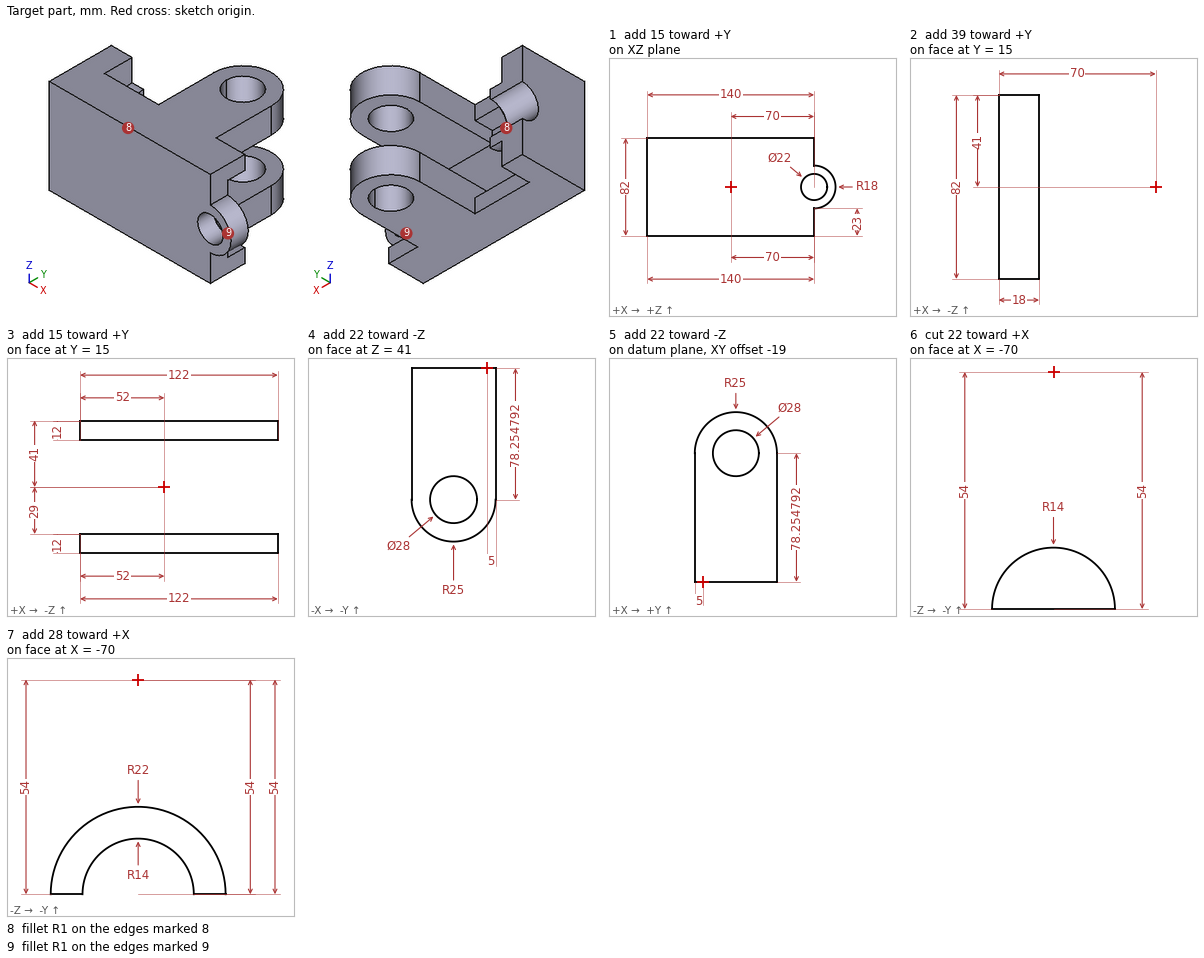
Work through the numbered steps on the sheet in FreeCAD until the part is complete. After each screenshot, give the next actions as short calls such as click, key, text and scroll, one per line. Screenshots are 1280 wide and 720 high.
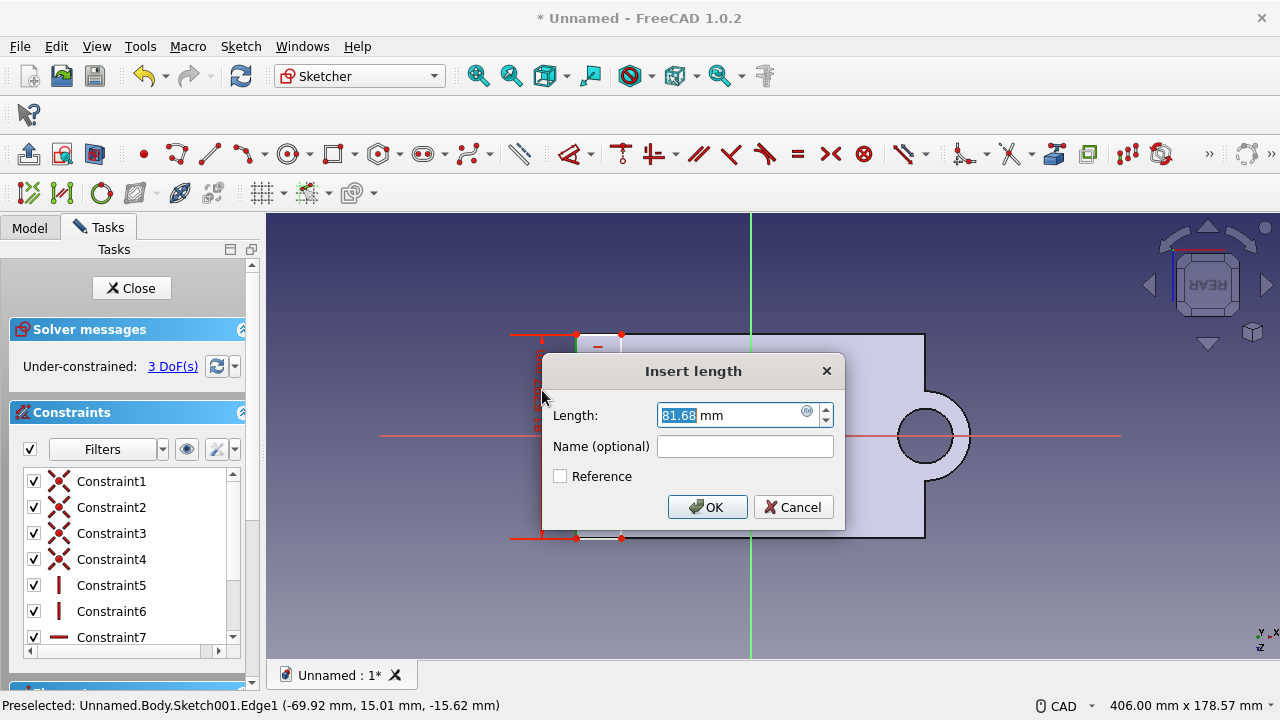
text(82)
key(Return)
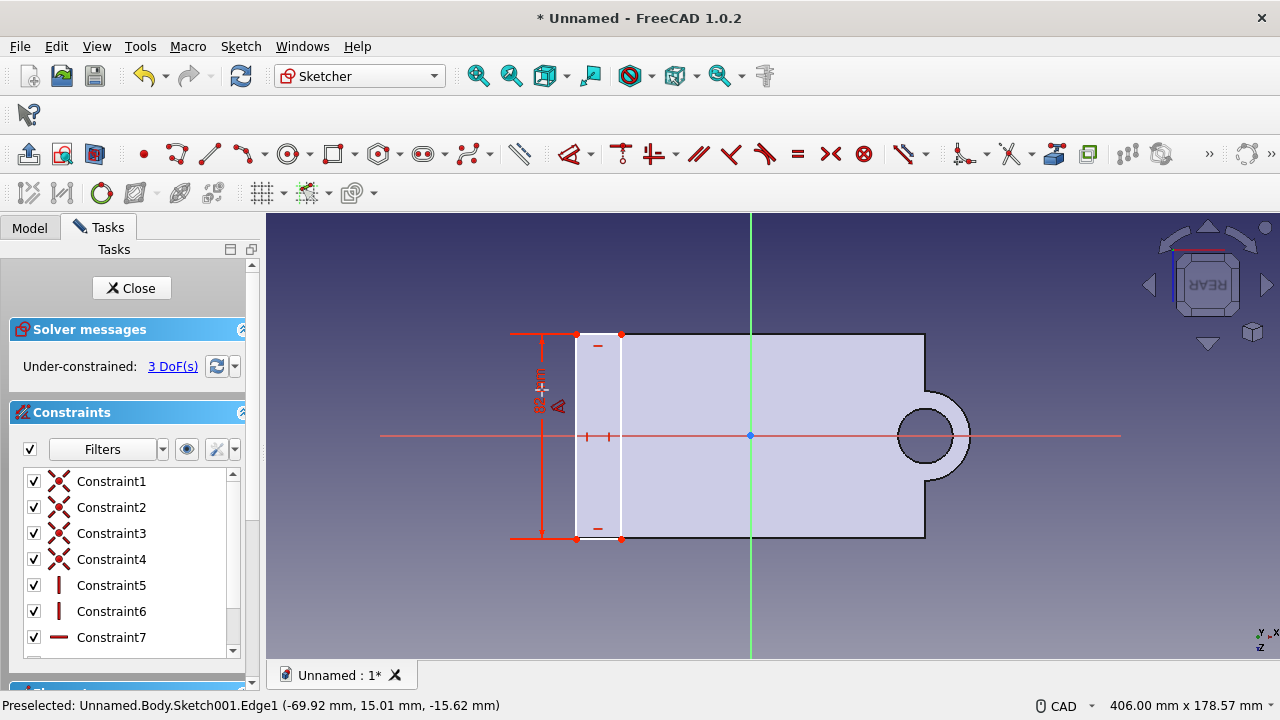
click(589, 539)
click(598, 573)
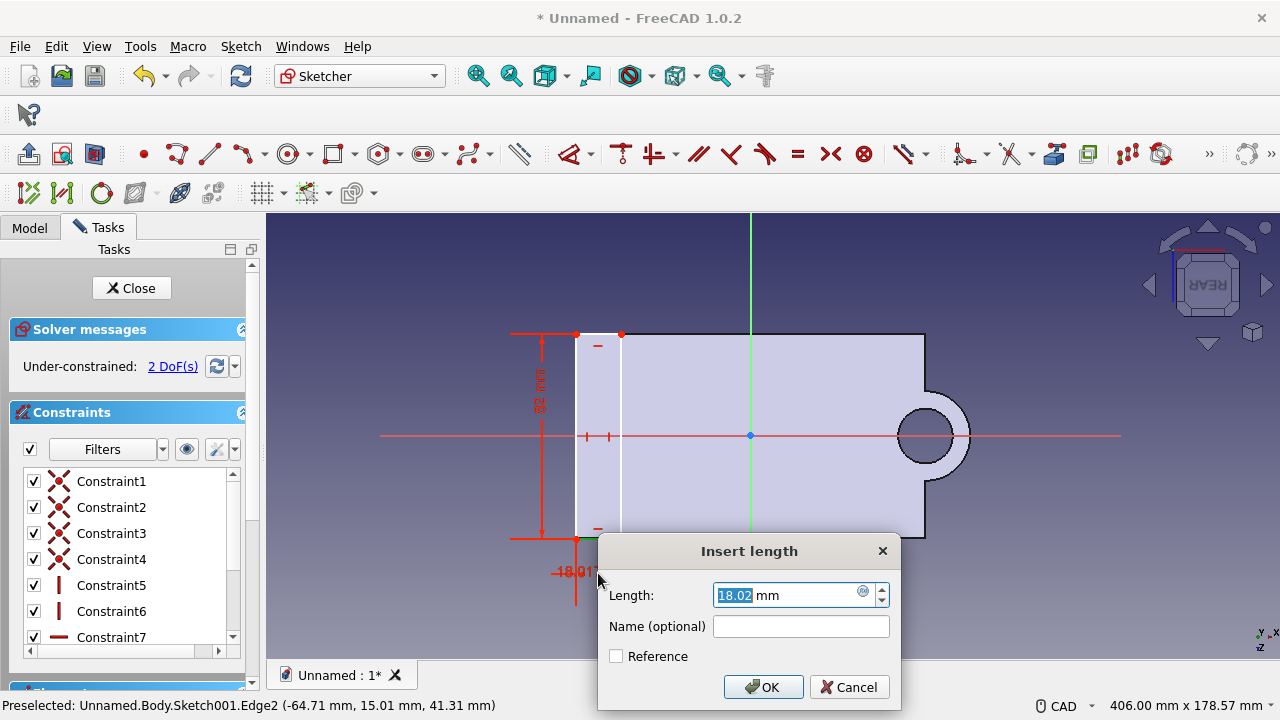
text(18)
key(Return)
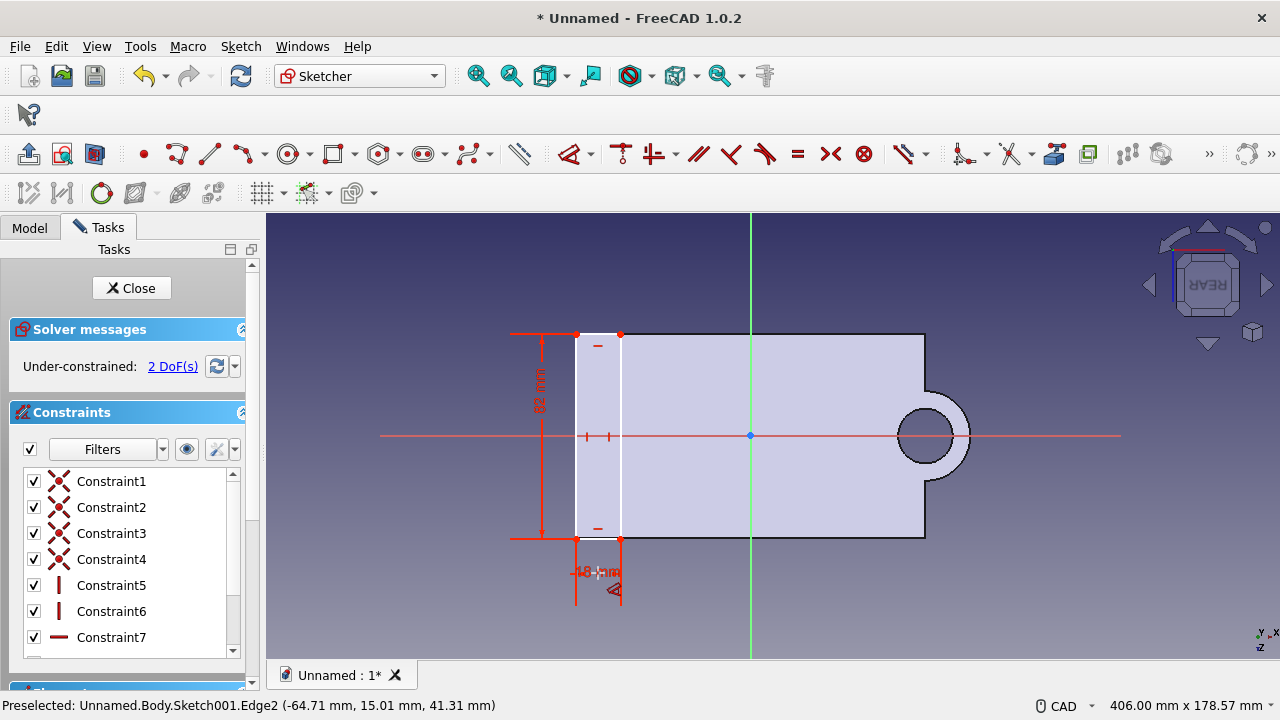
click(576, 334)
click(663, 300)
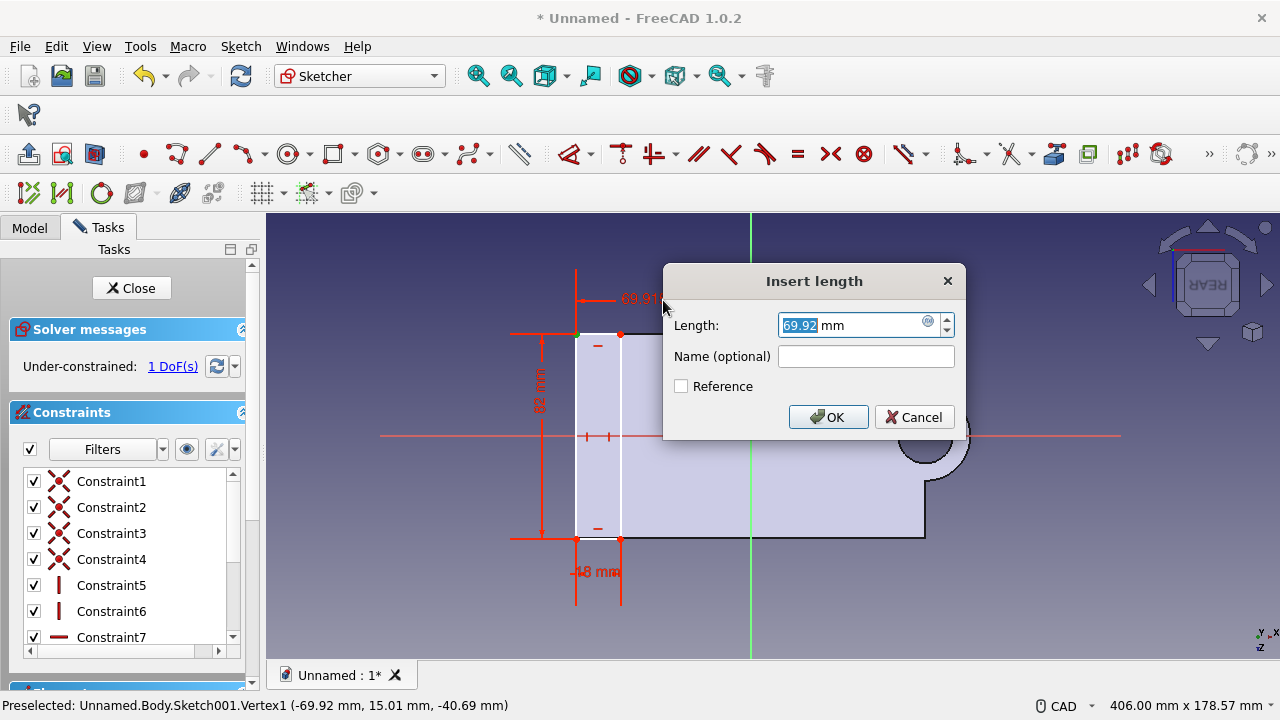
text(70)
key(Return)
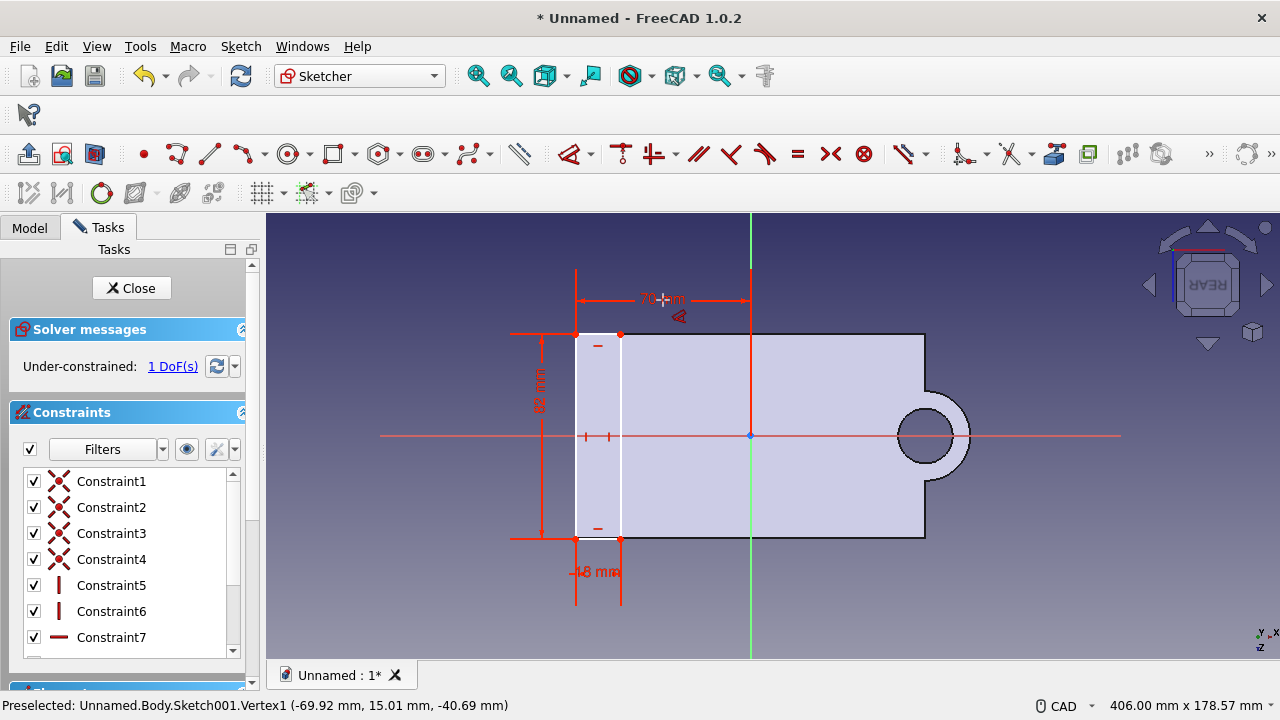
click(576, 334)
click(785, 385)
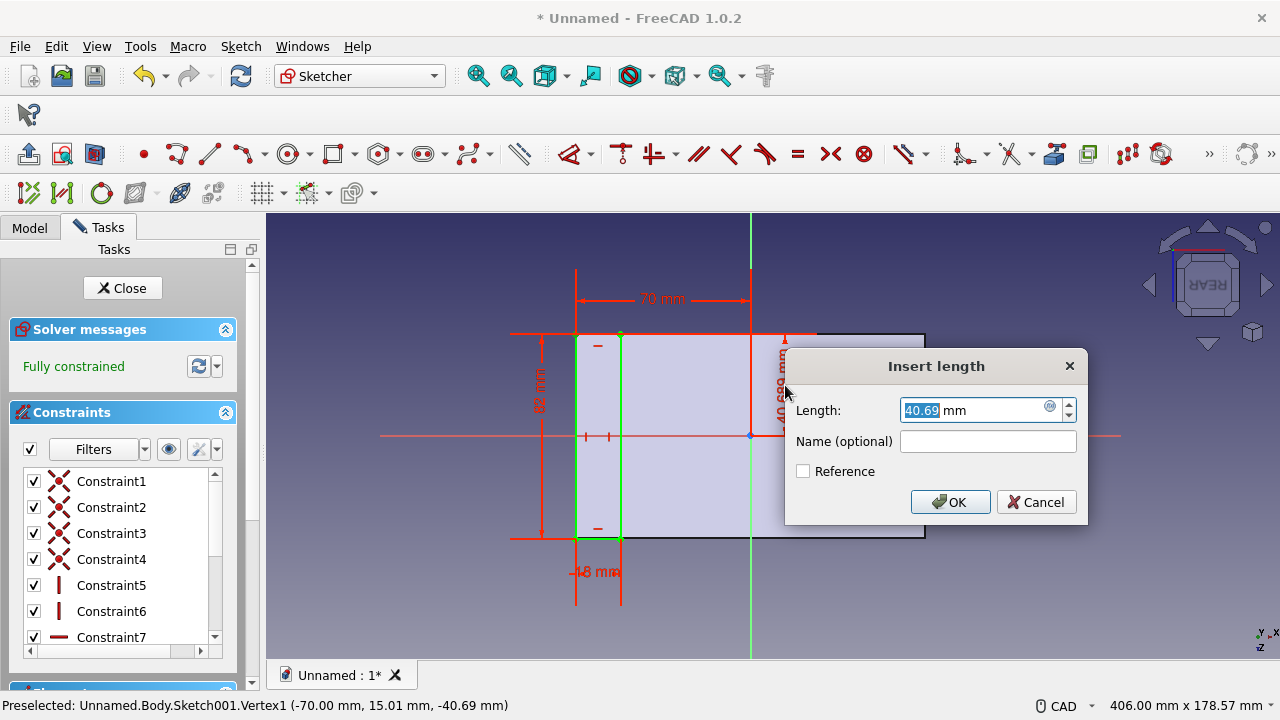
text(41)
key(Return)
key(Escape)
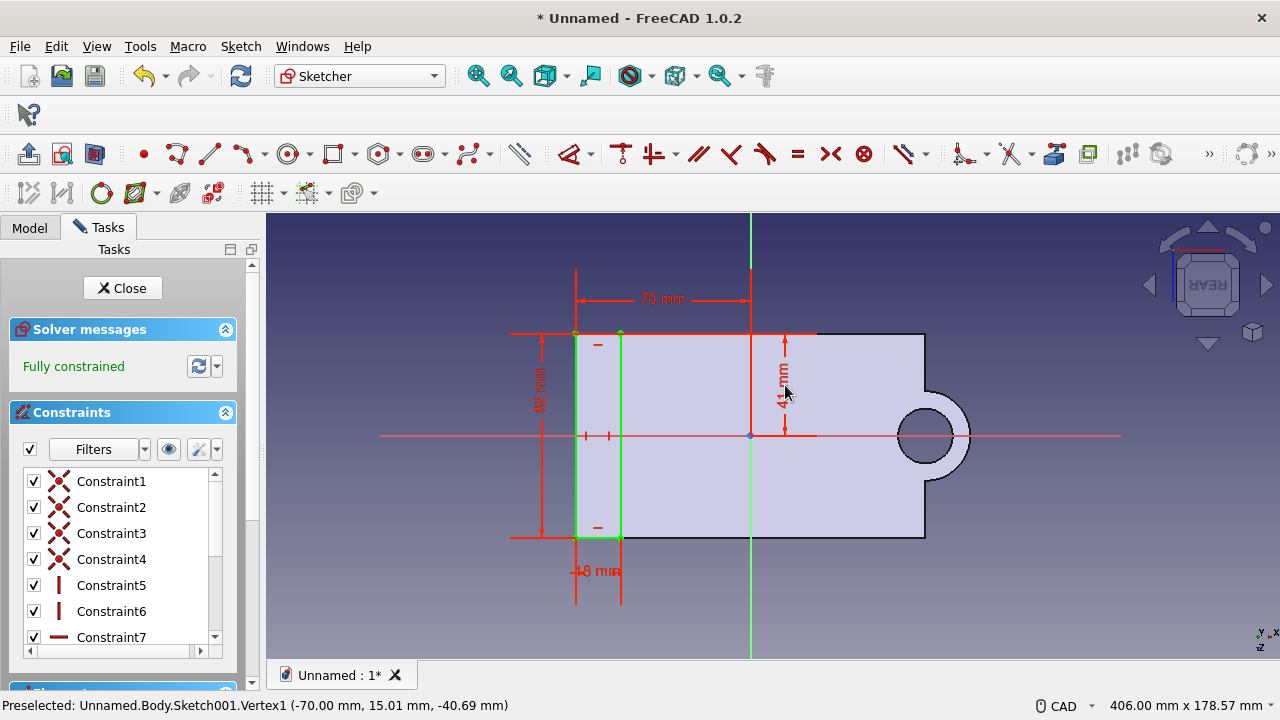
click(123, 288)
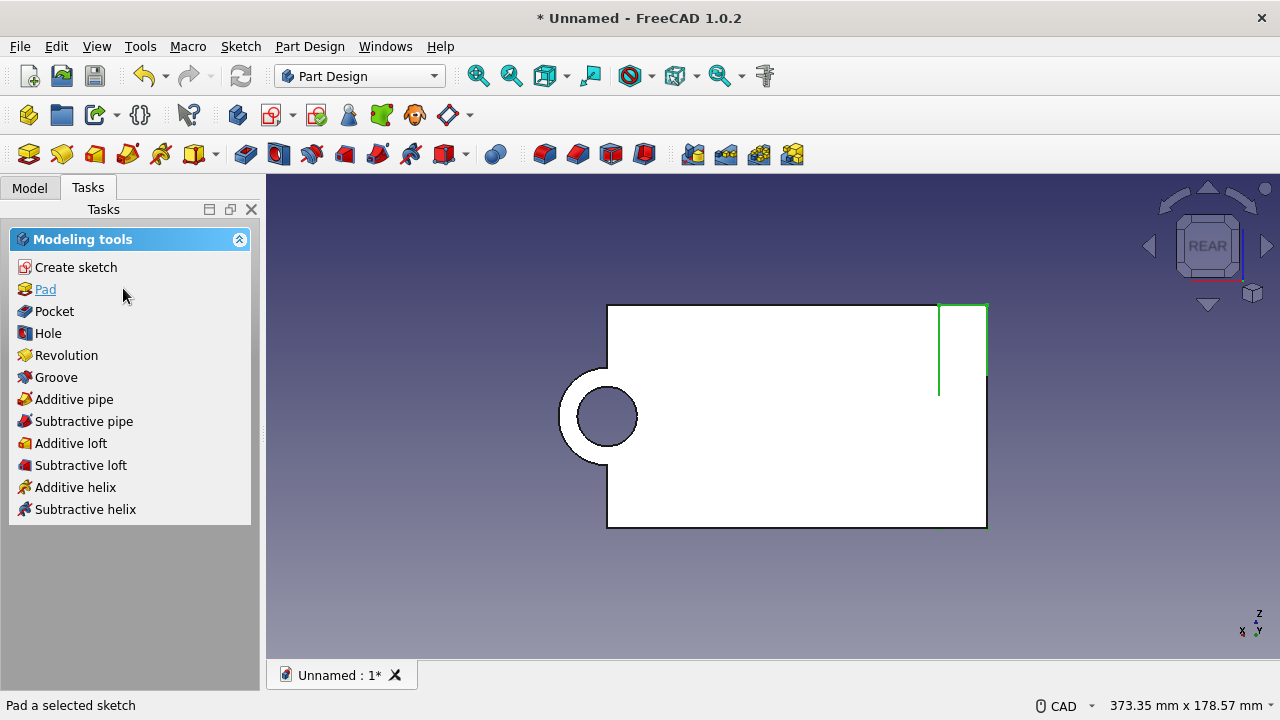
click(29, 154)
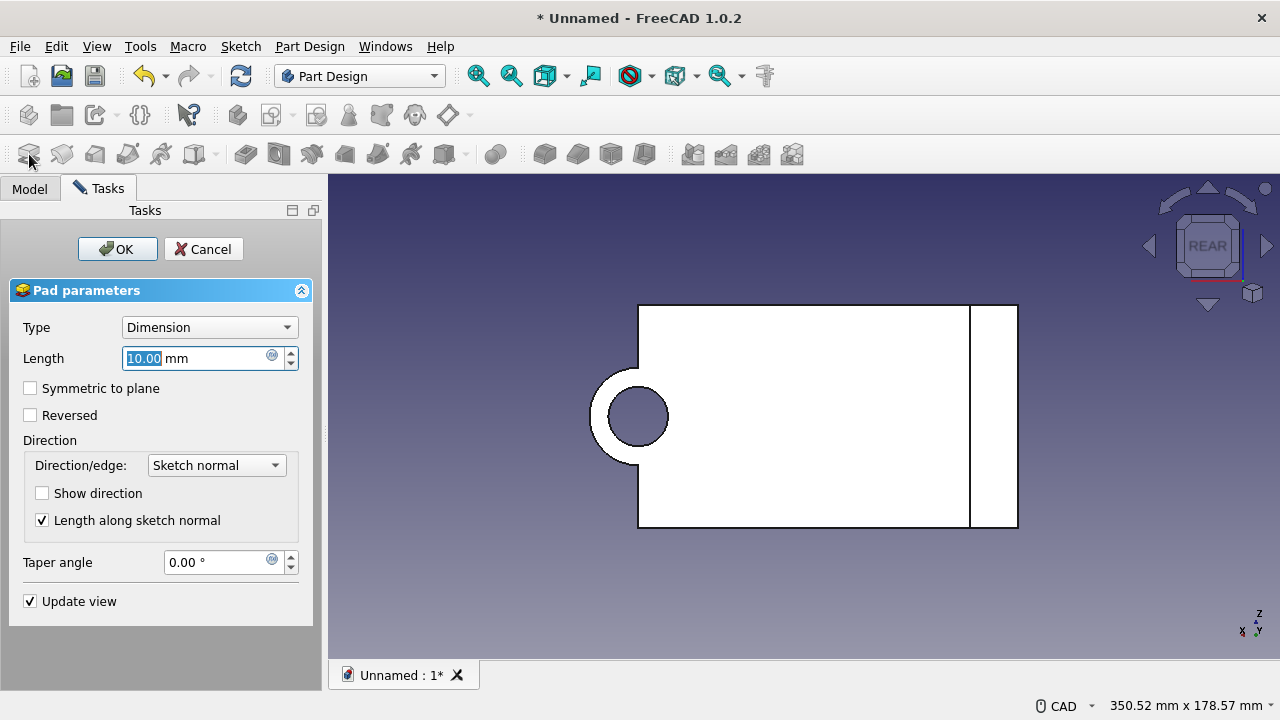
text(39)
key(Tab)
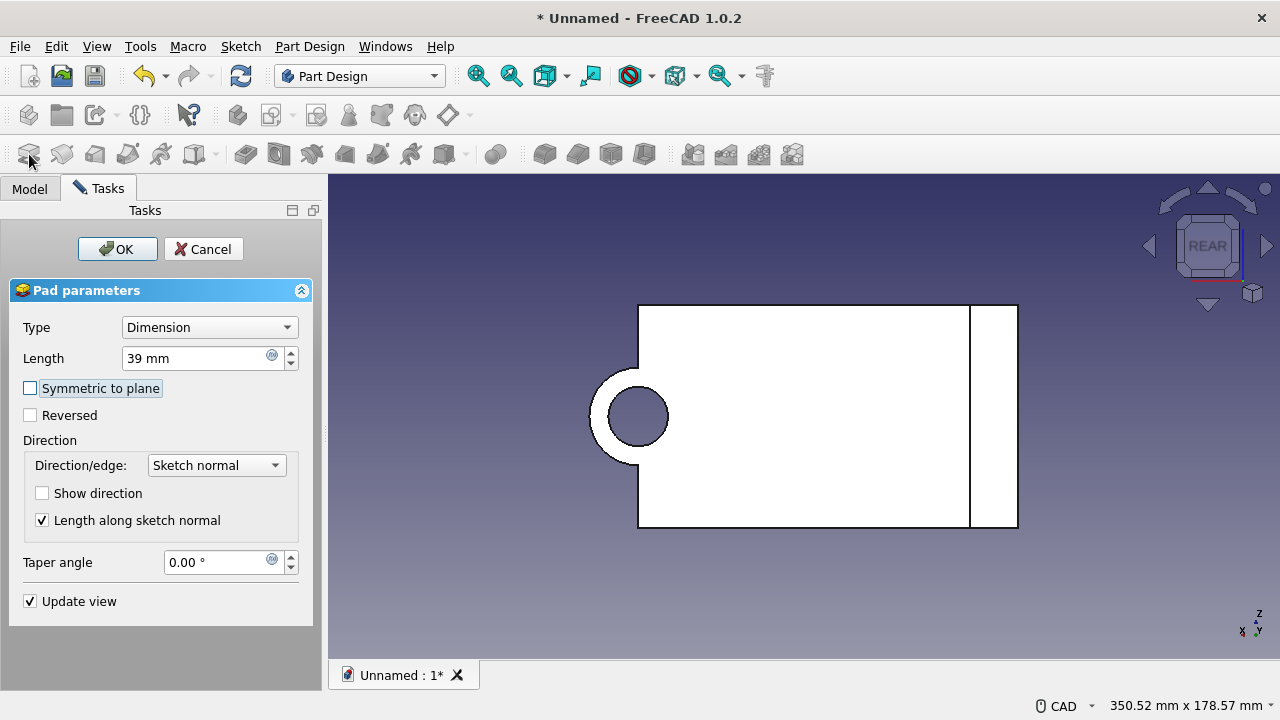
click(118, 249)